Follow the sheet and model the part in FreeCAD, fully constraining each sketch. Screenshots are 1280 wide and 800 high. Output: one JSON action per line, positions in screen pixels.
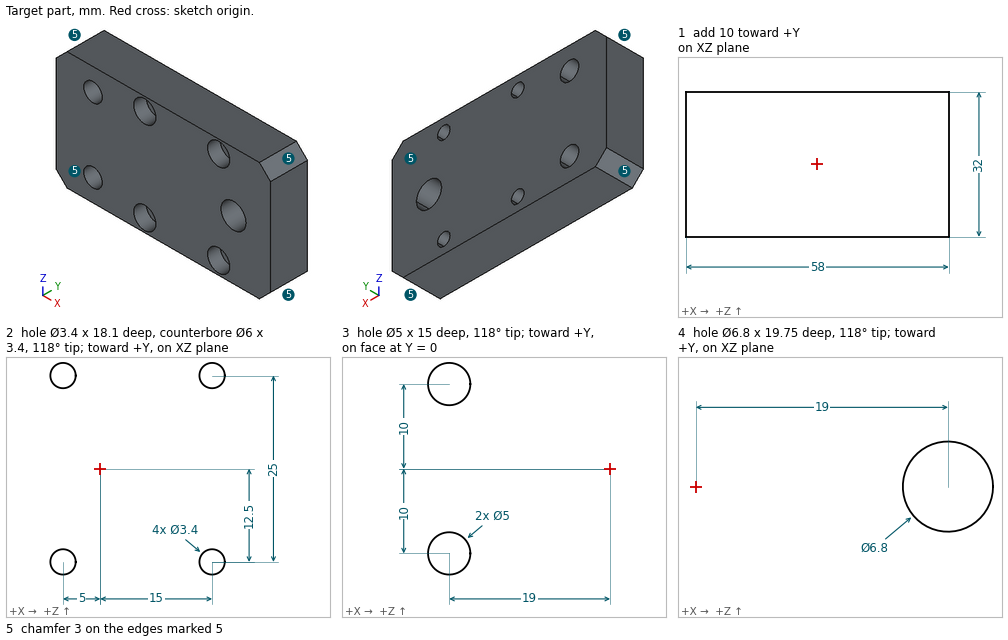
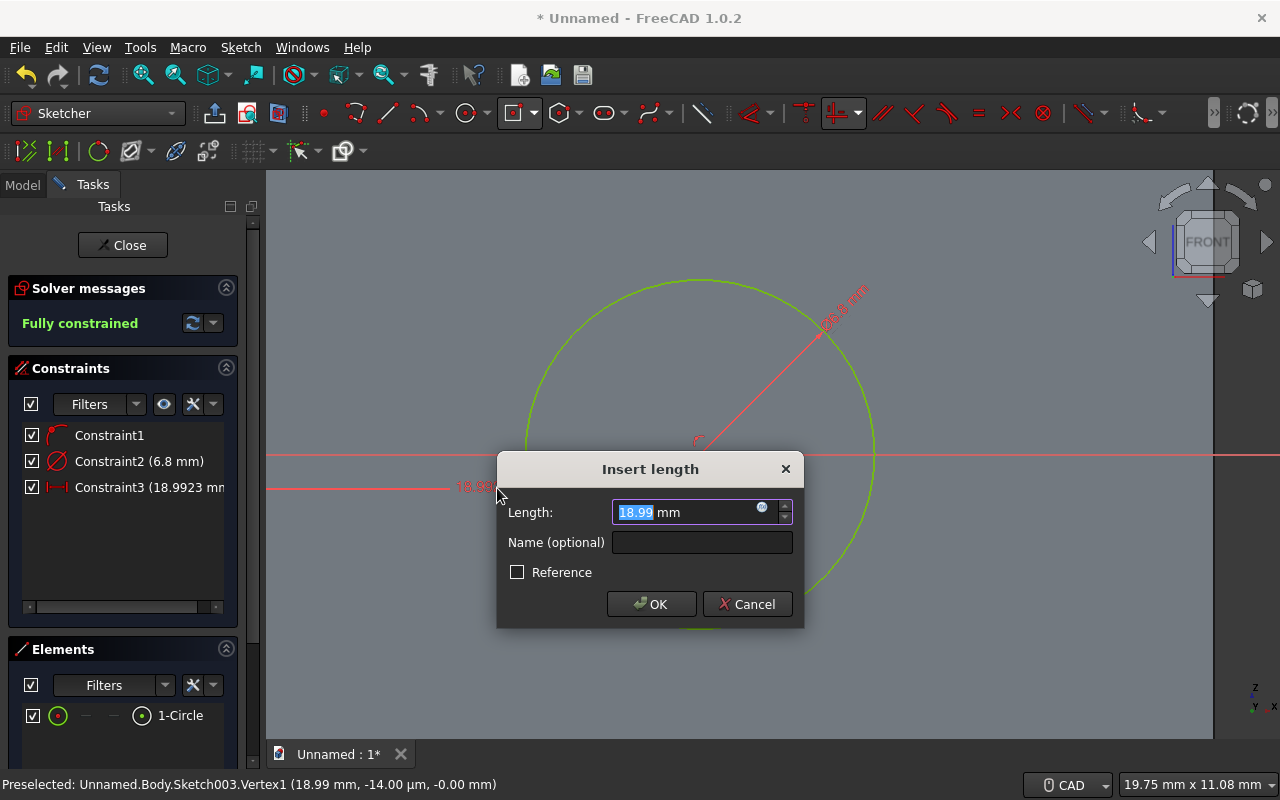
{"action": "type", "text": "19"}
{"action": "key", "text": "Return"}
{"action": "key", "text": "Escape"}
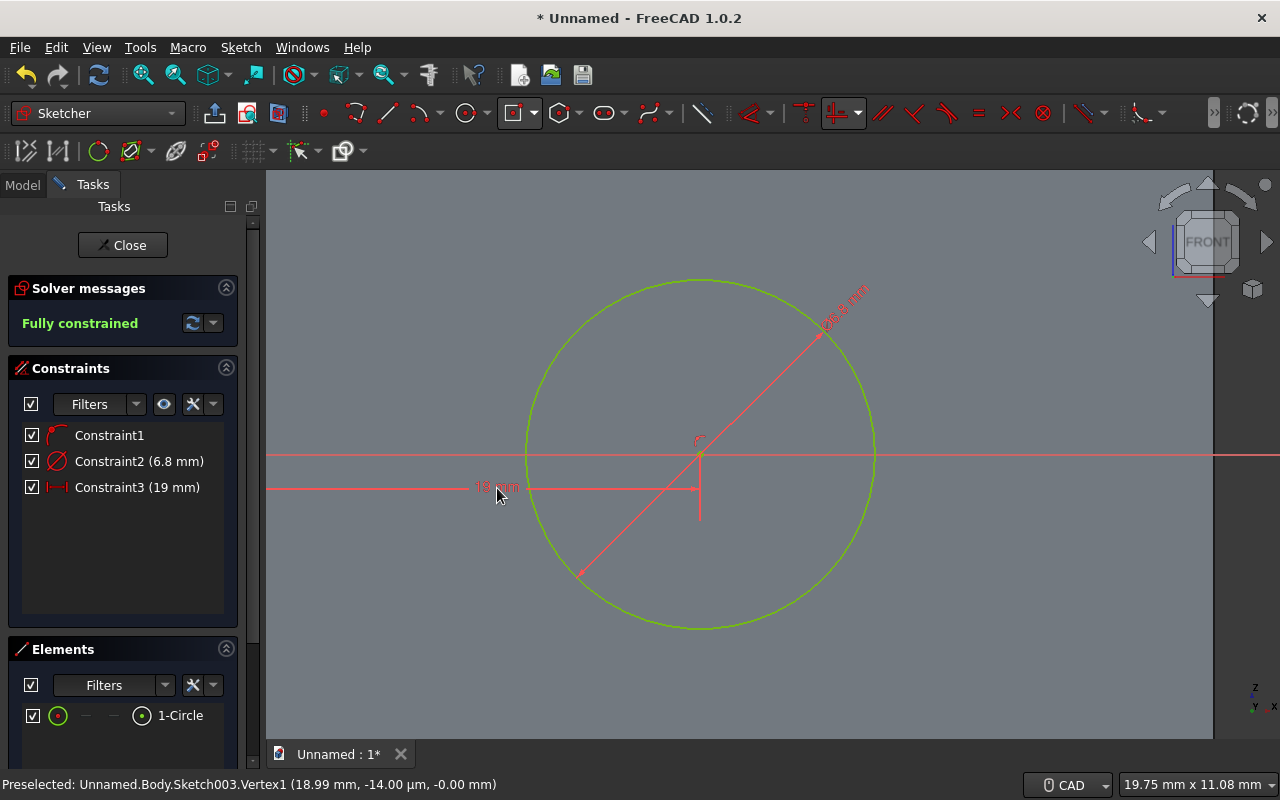
{"action": "left_click", "coordinate": [123, 245]}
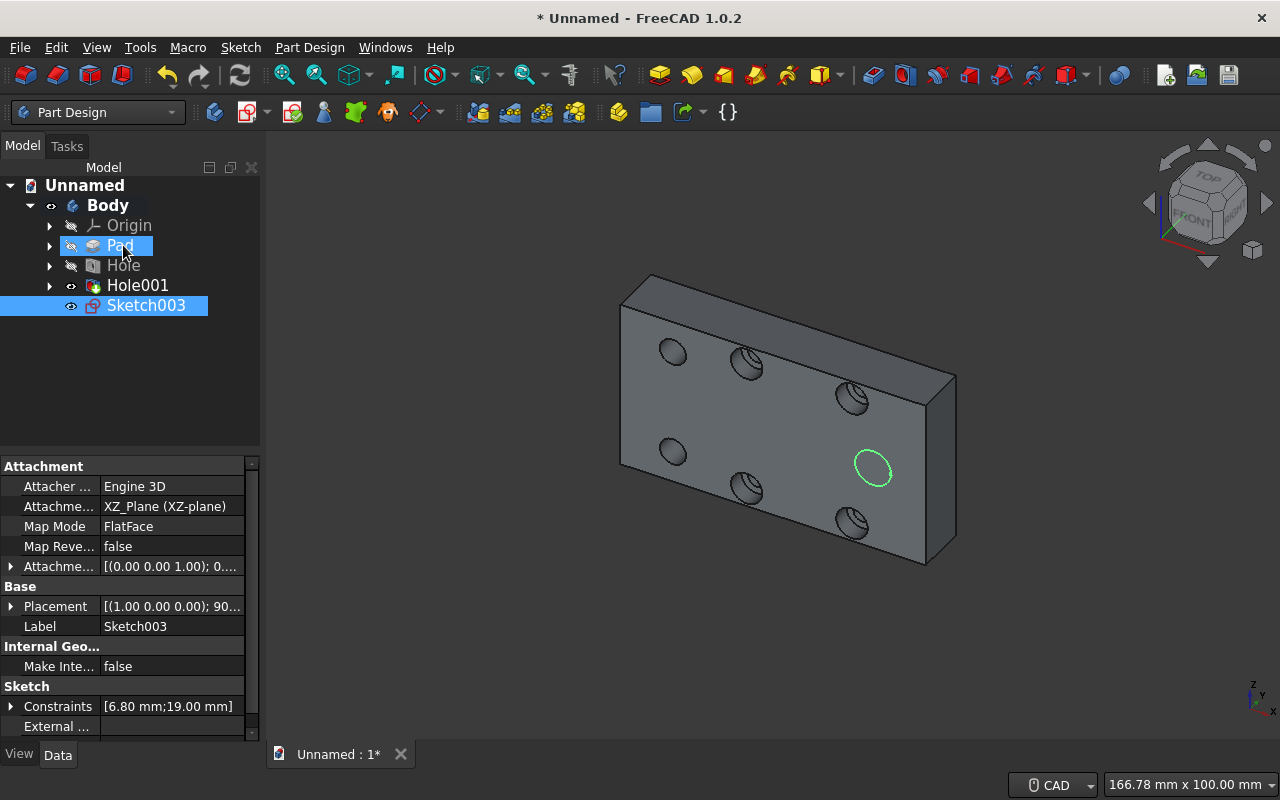
{"action": "left_click", "coordinate": [906, 76]}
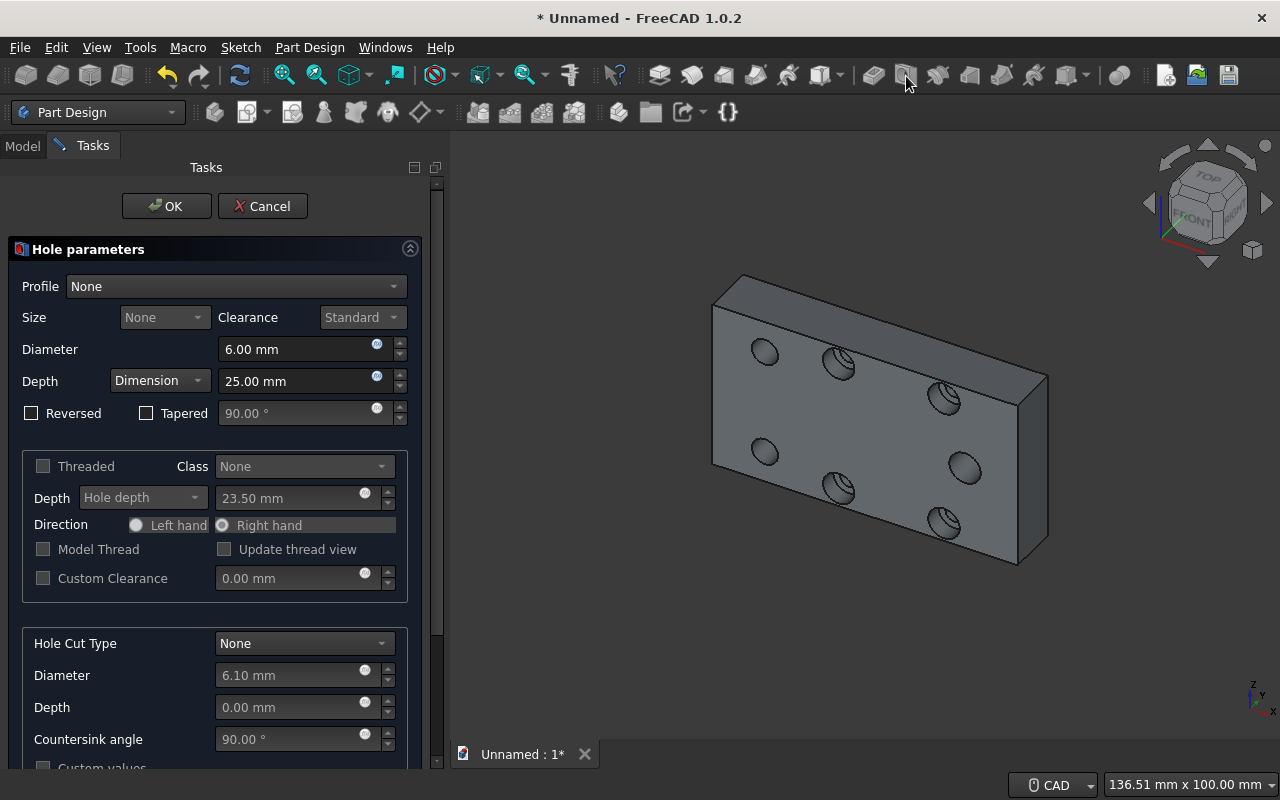
{"action": "triple_click", "coordinate": [305, 349]}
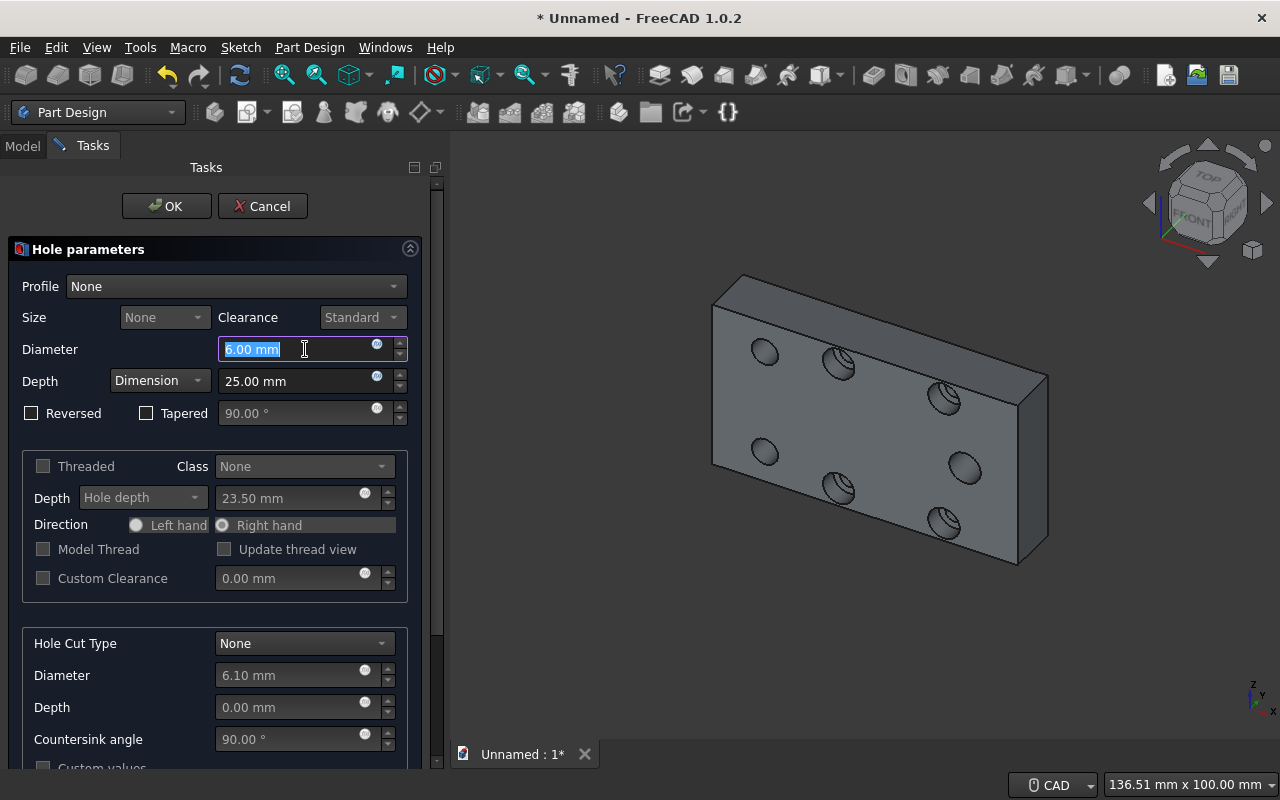
{"action": "type", "text": "6.8"}
{"action": "key", "text": "Tab"}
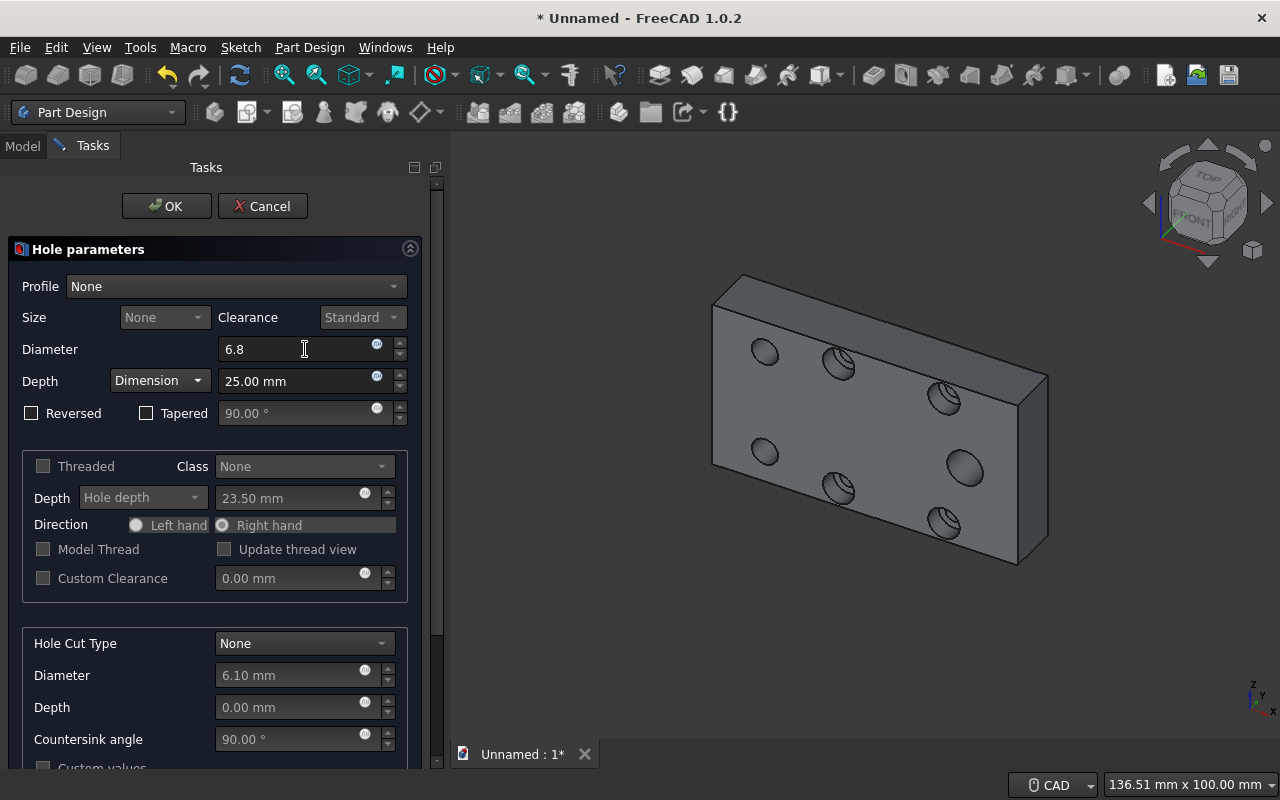
{"action": "triple_click", "coordinate": [305, 381]}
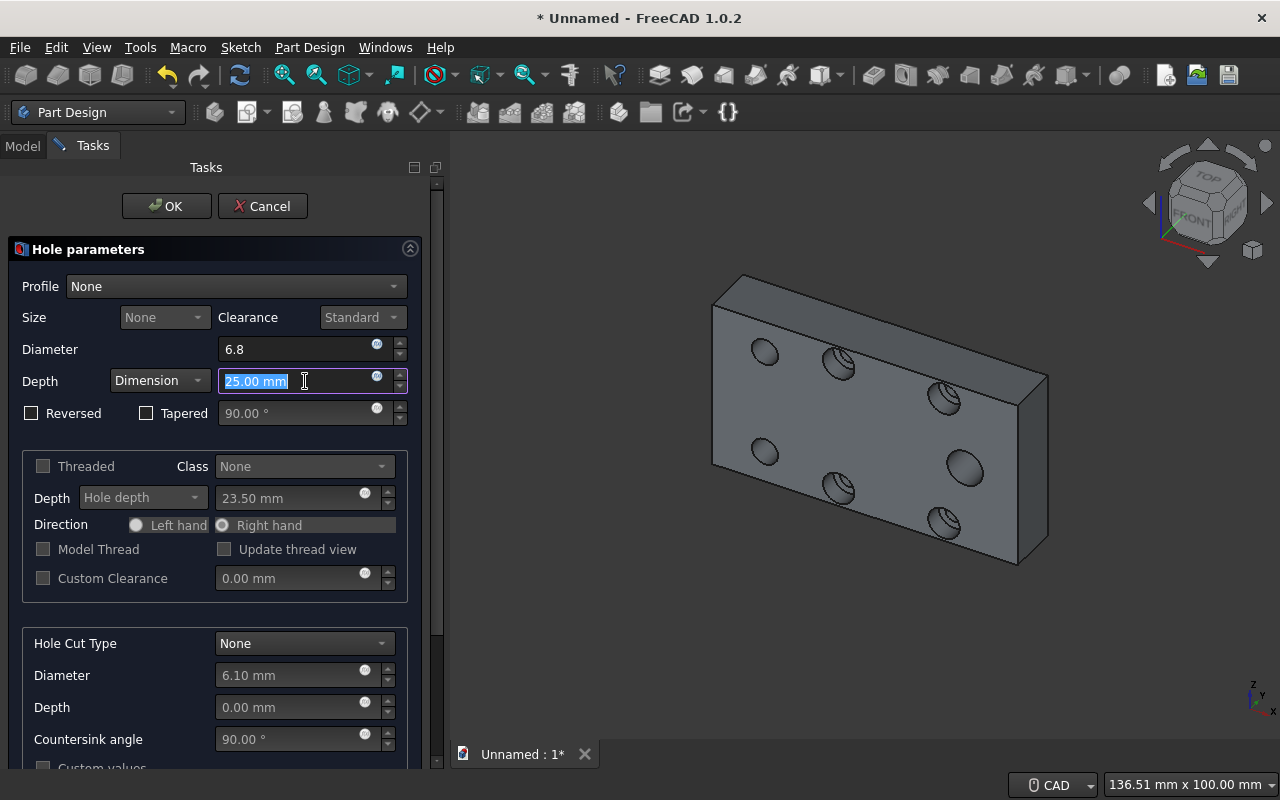
{"action": "type", "text": "19.75"}
{"action": "key", "text": "Tab"}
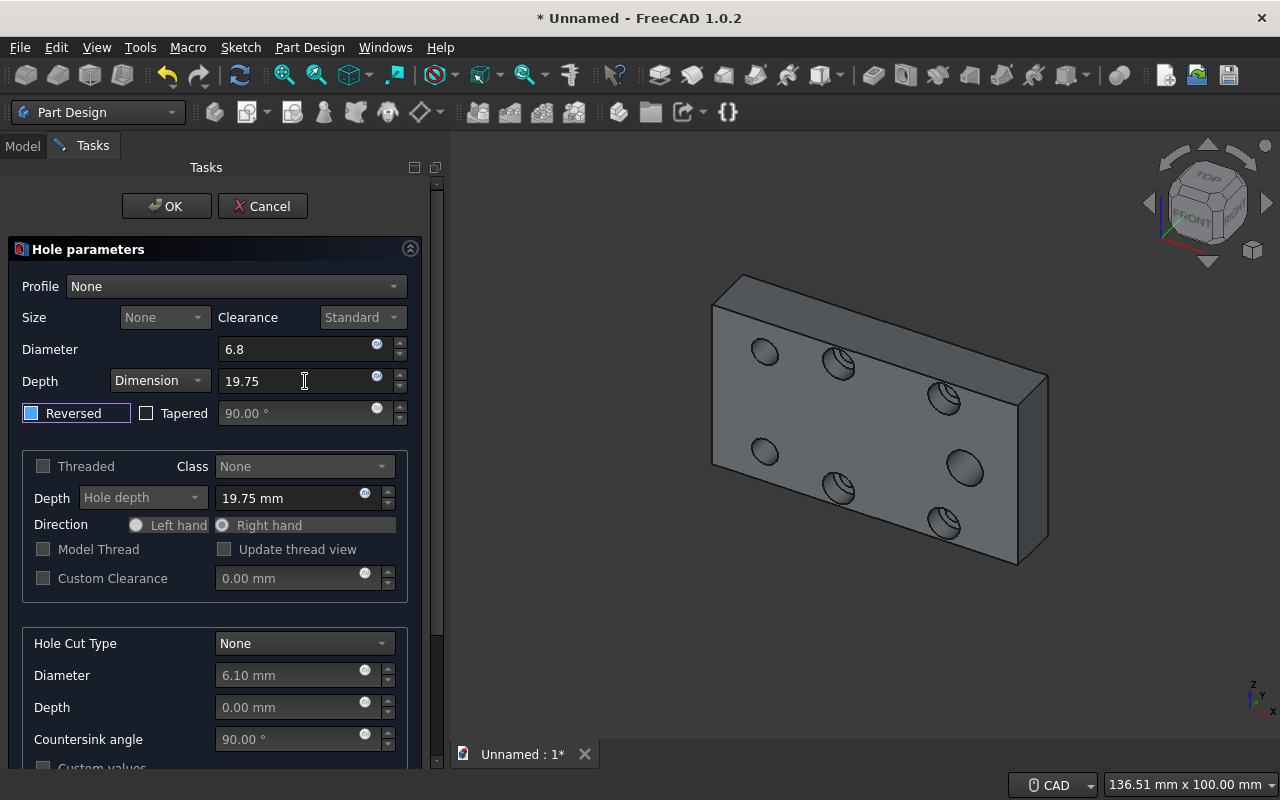
{"action": "left_click", "coordinate": [167, 206]}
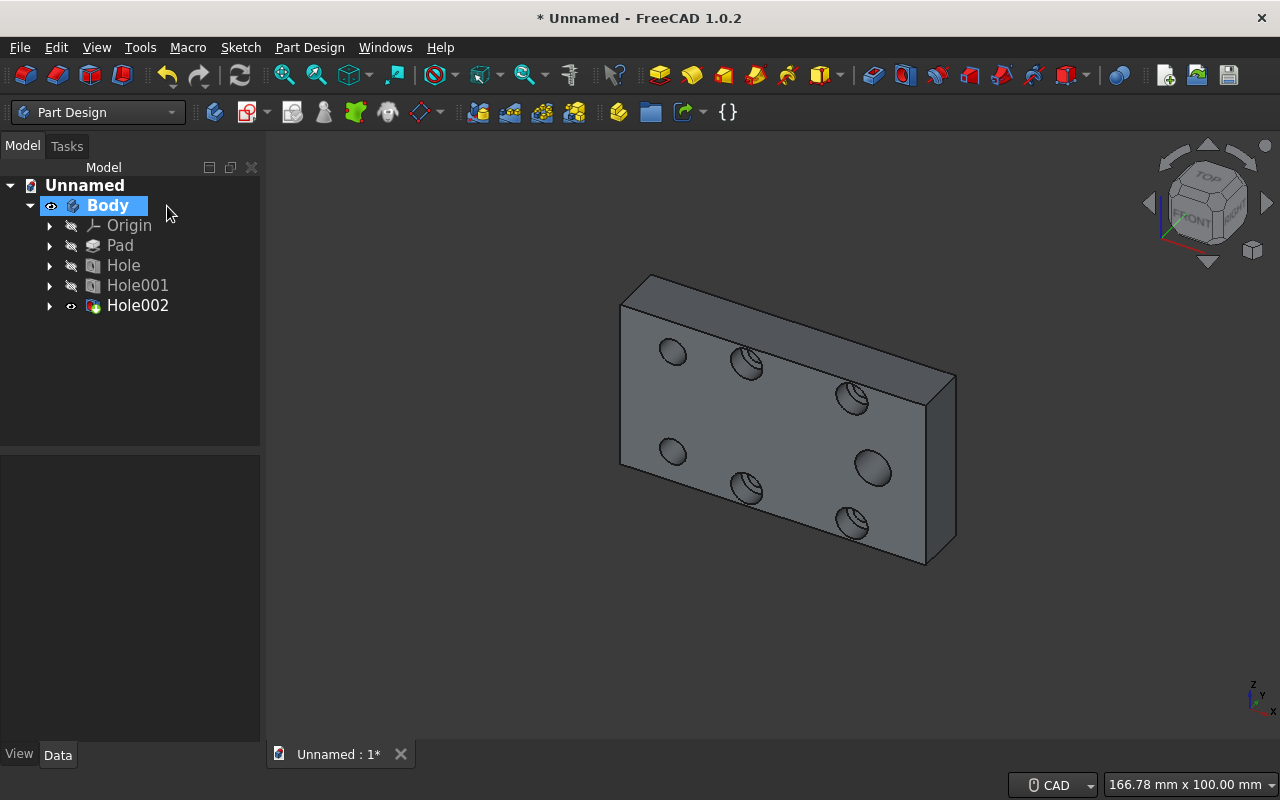
{"action": "left_click", "coordinate": [941, 390]}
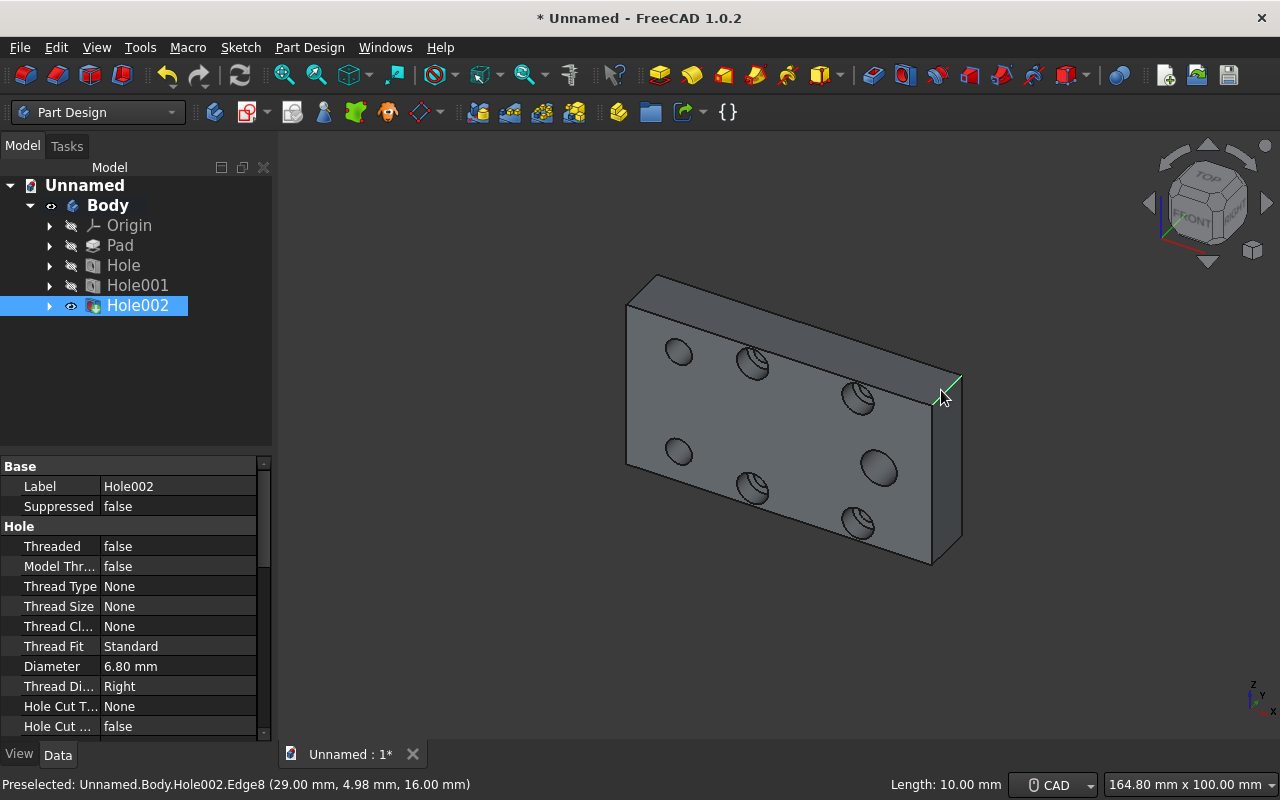
{"action": "key", "text": "0"}